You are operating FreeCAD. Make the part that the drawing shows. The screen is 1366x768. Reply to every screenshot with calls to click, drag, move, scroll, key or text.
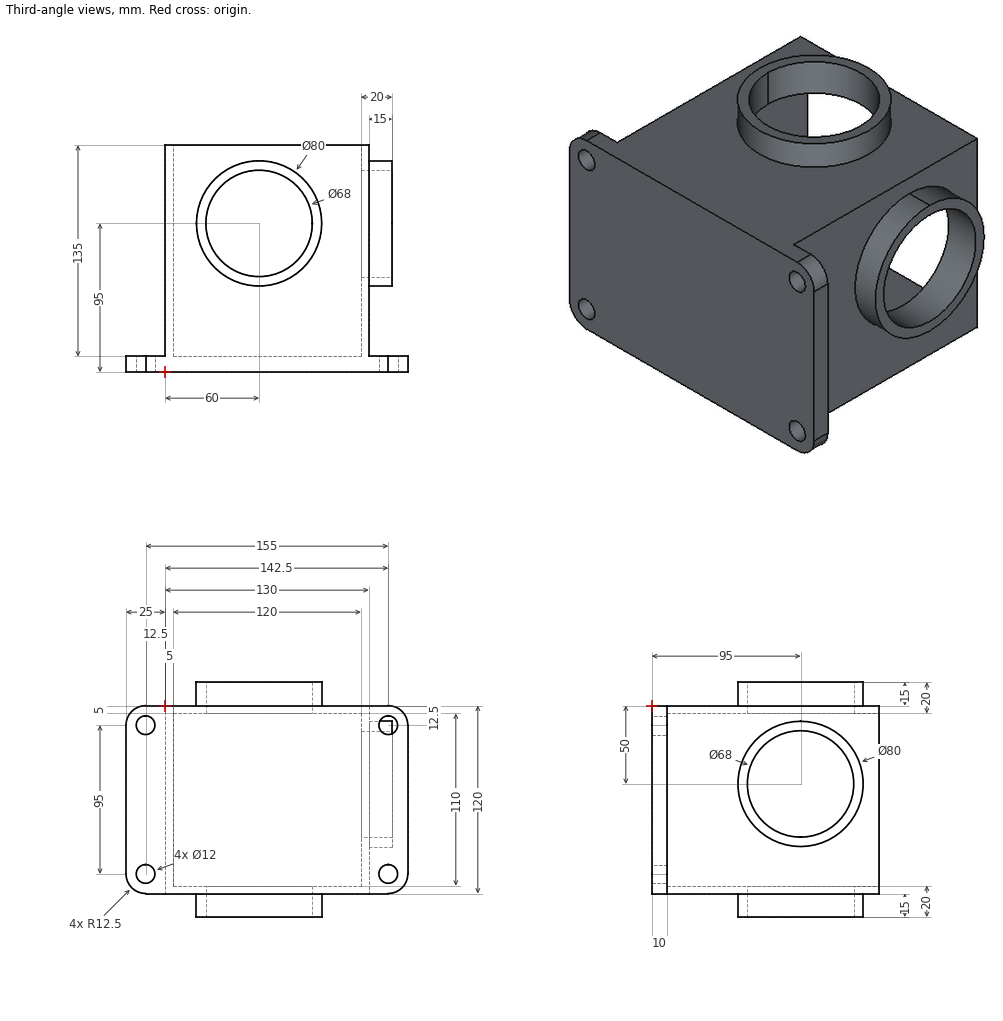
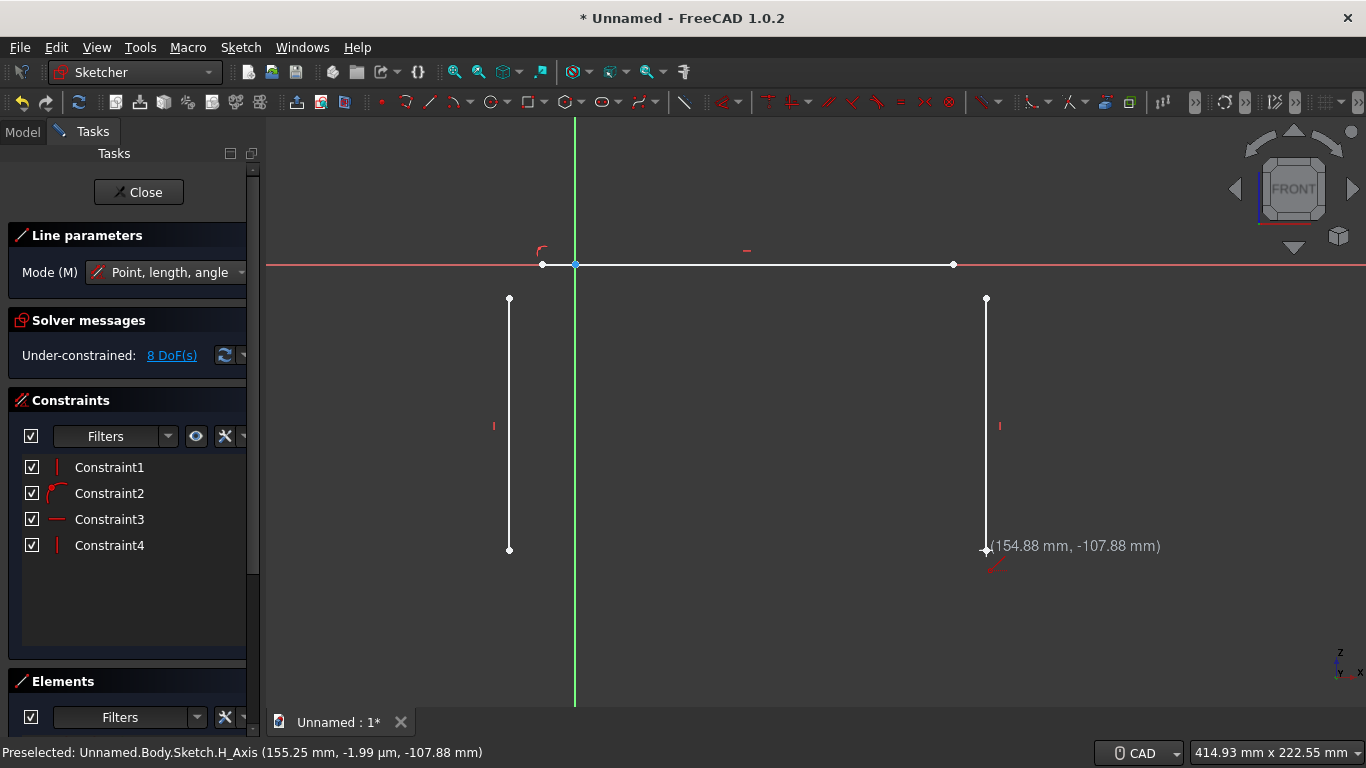
click(953, 583)
click(542, 583)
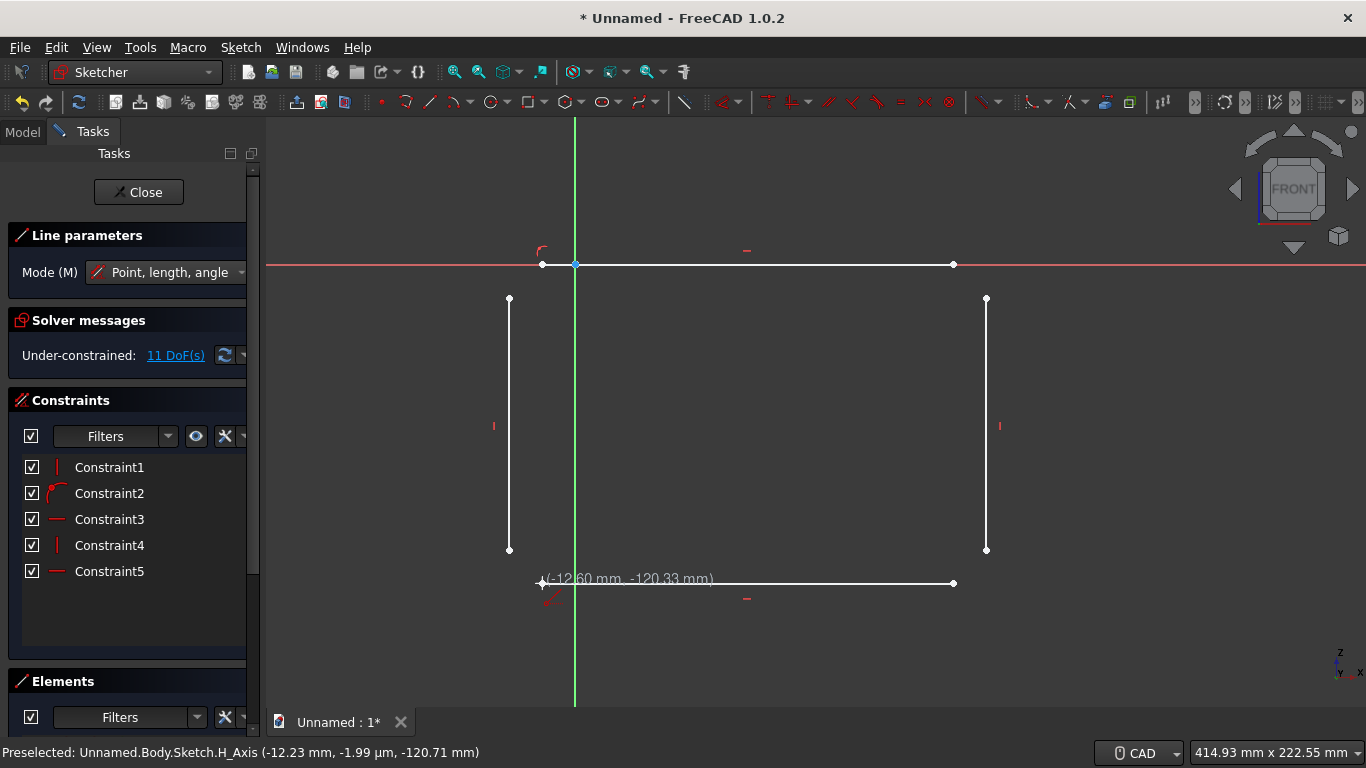
click(472, 102)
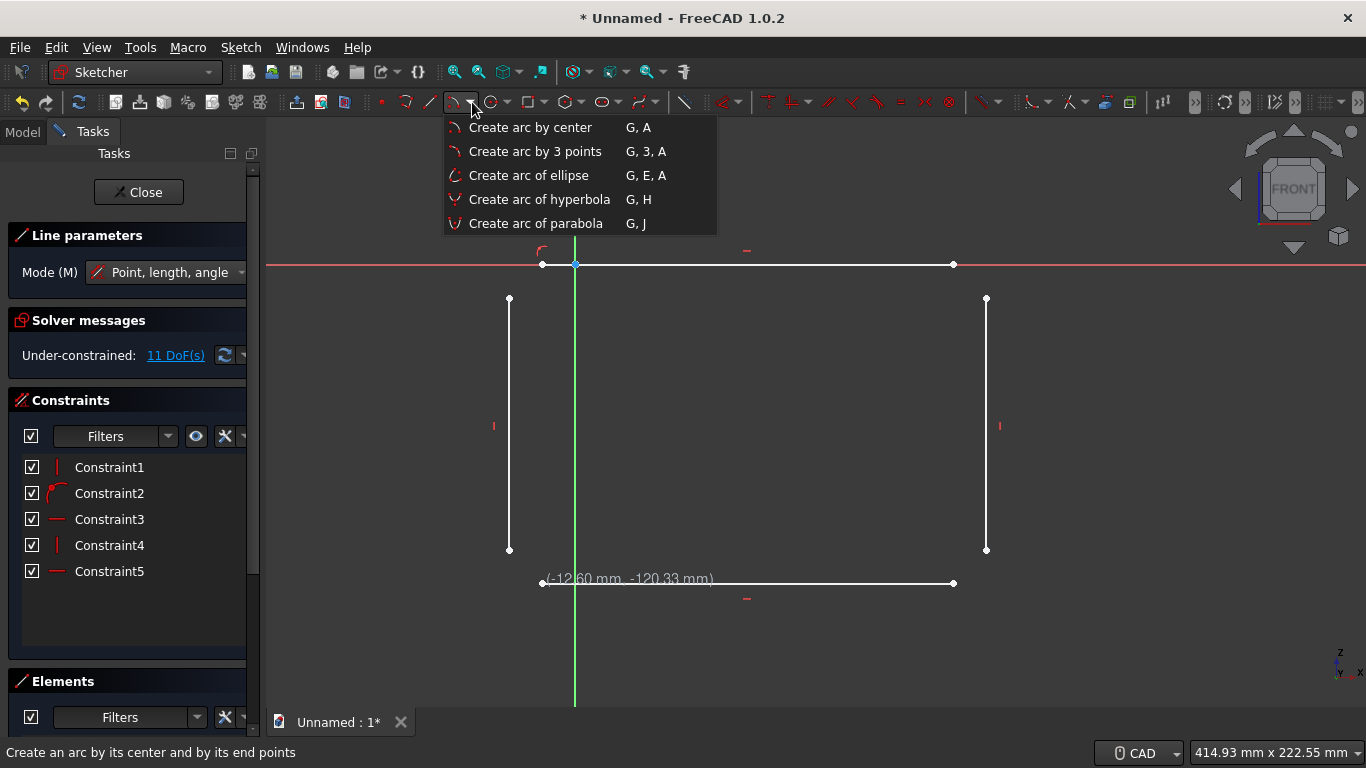
click(580, 151)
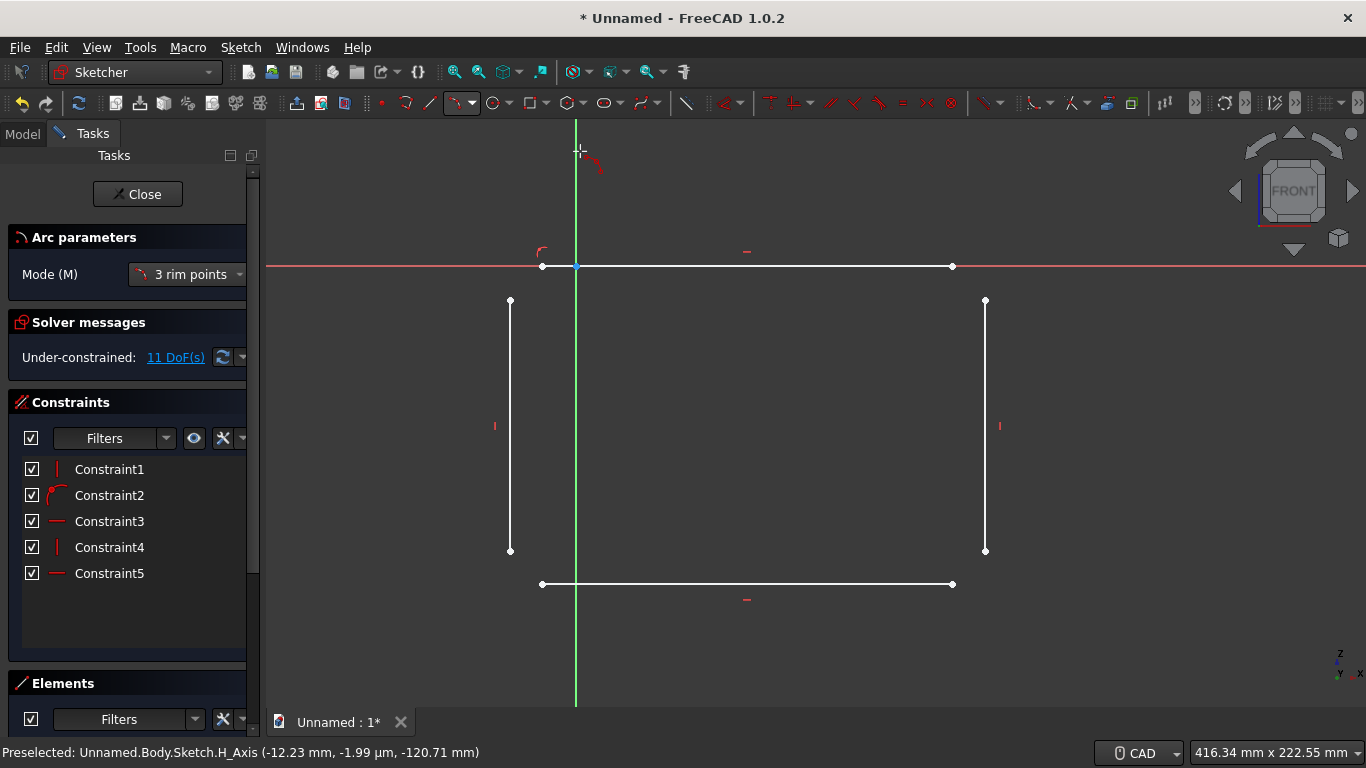
click(510, 300)
click(543, 266)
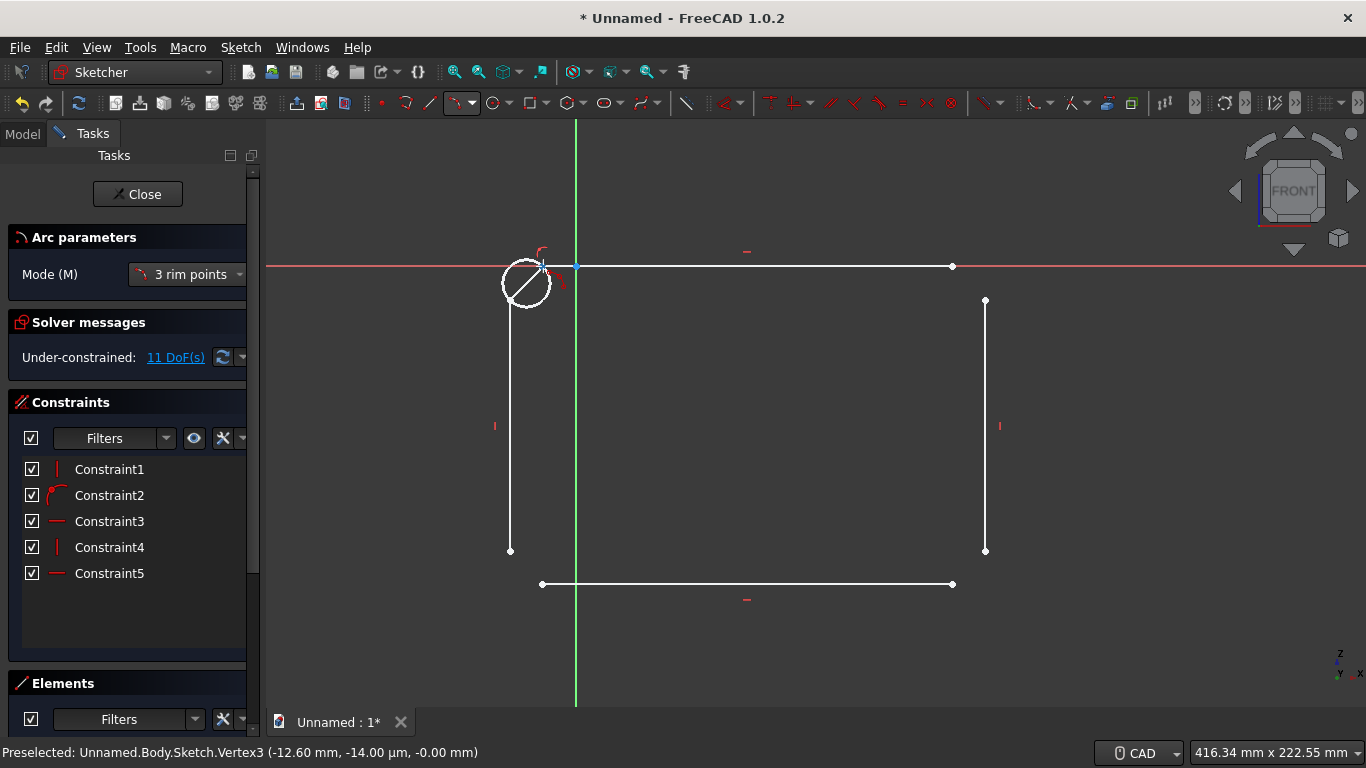
scroll(520, 276, up, 3)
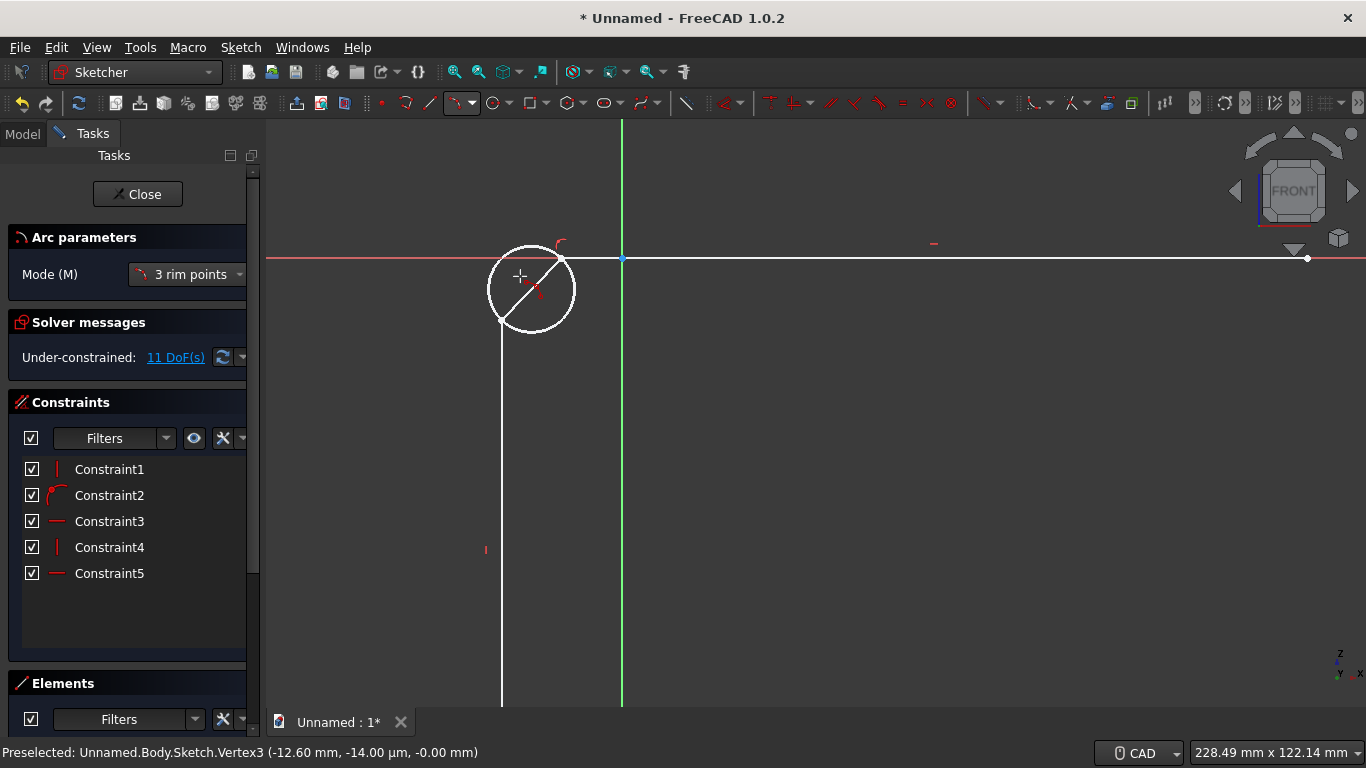
click(520, 276)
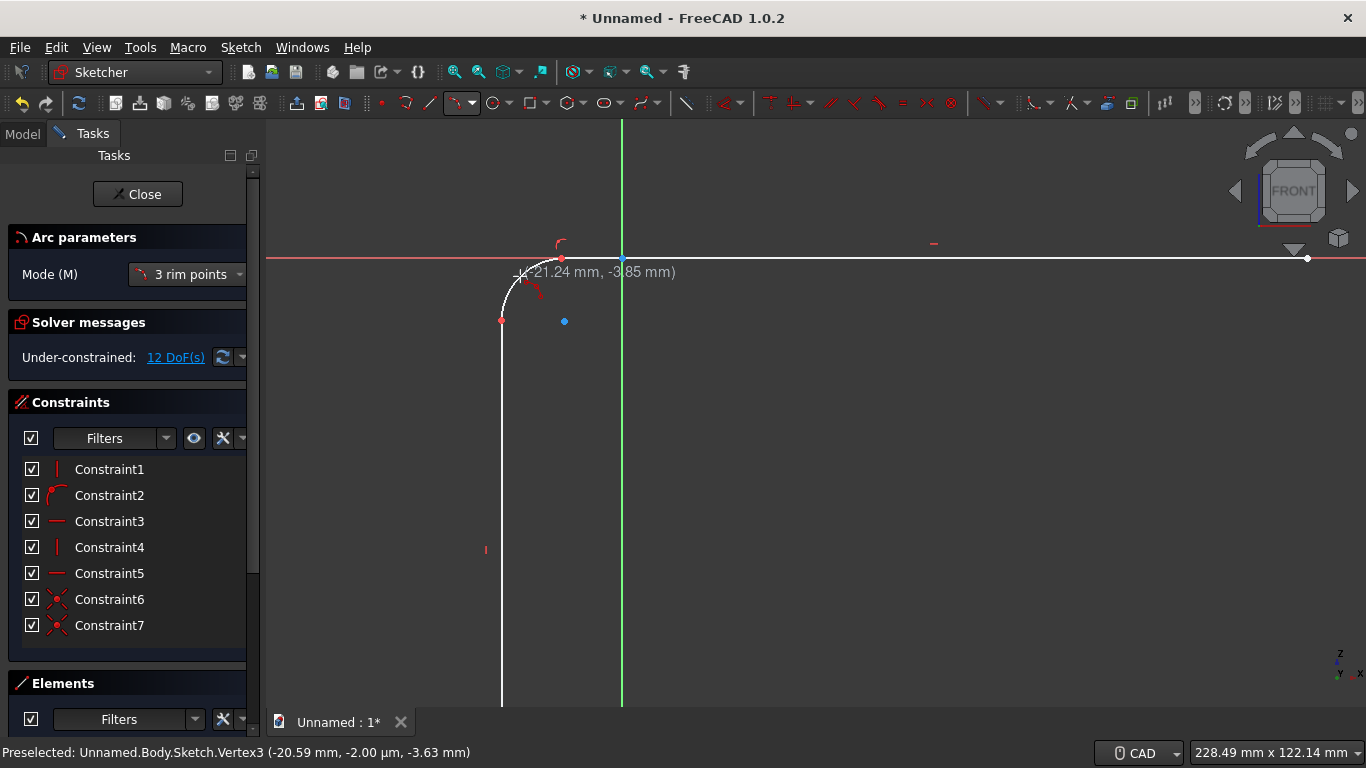
scroll(366, 147, down, 2)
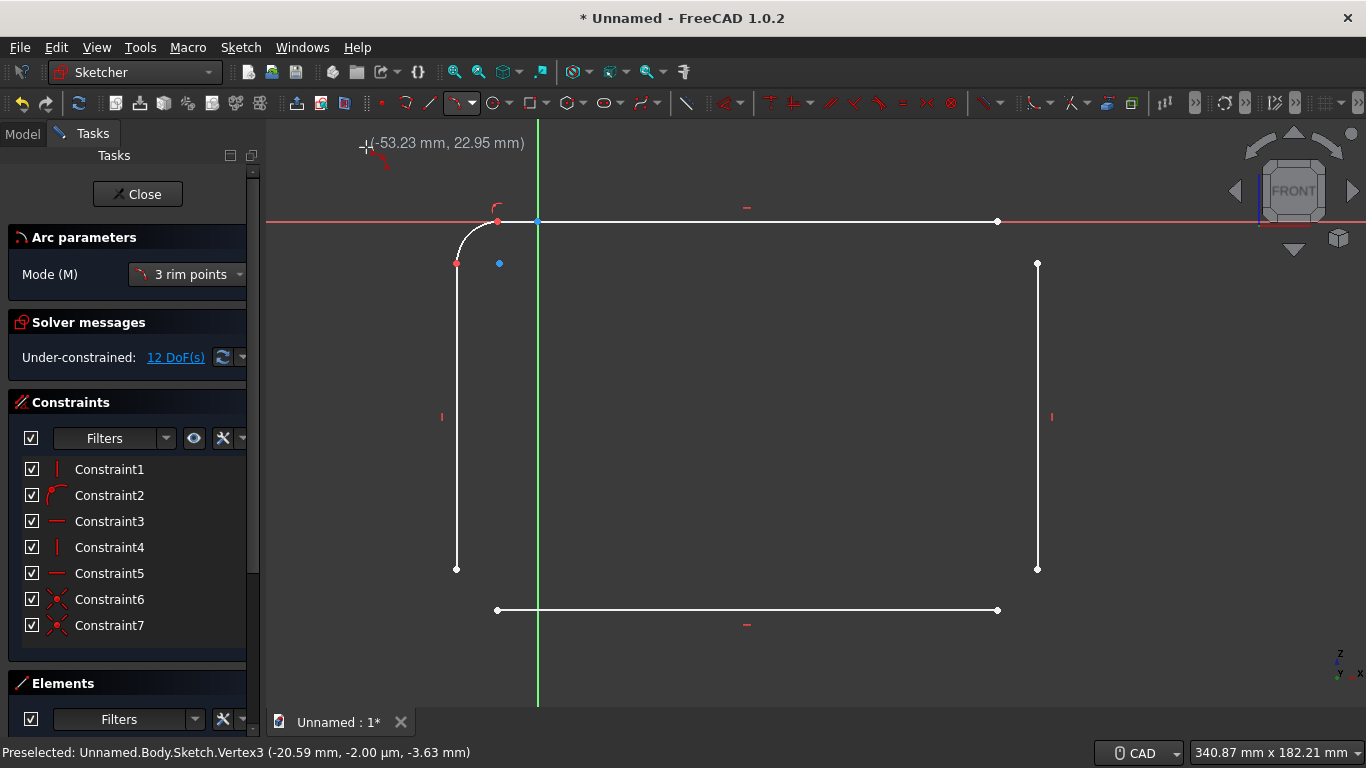
click(997, 233)
click(1038, 263)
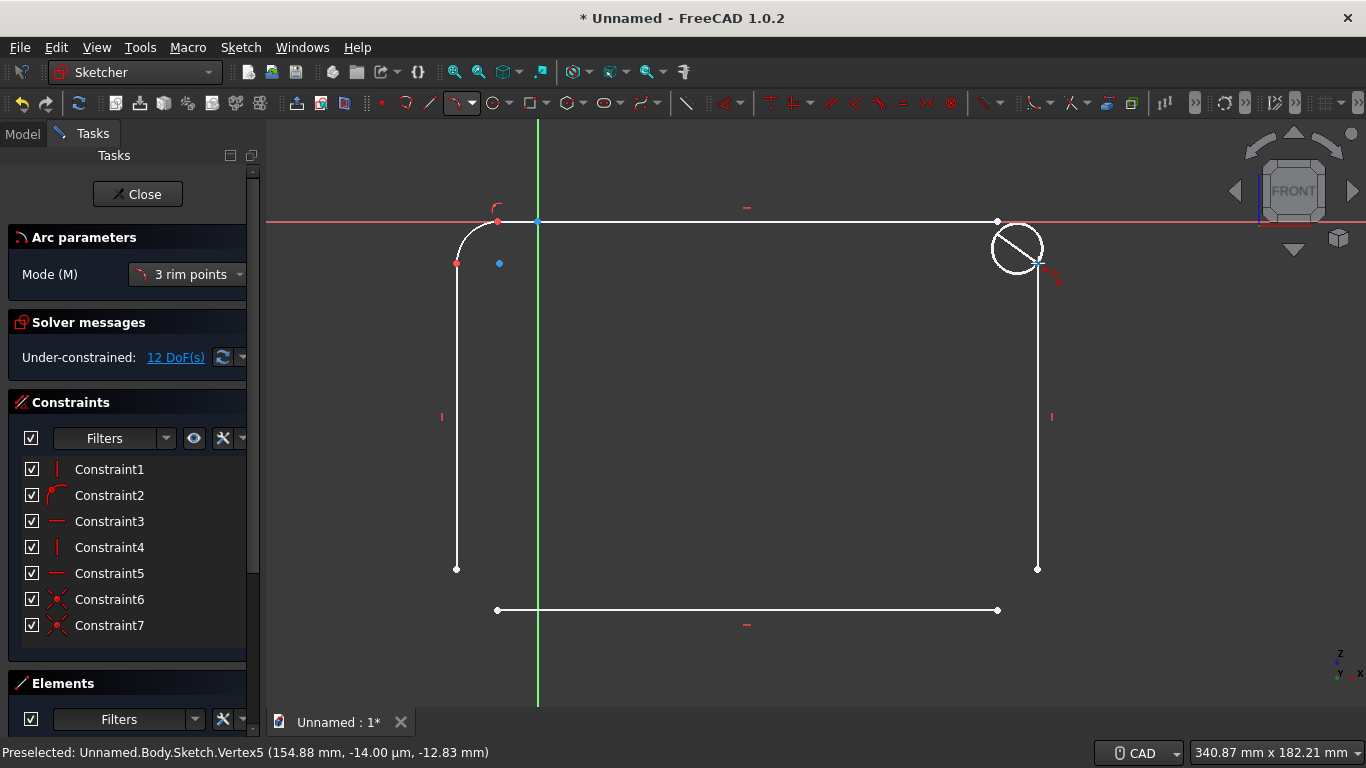
scroll(1026, 234, up, 2)